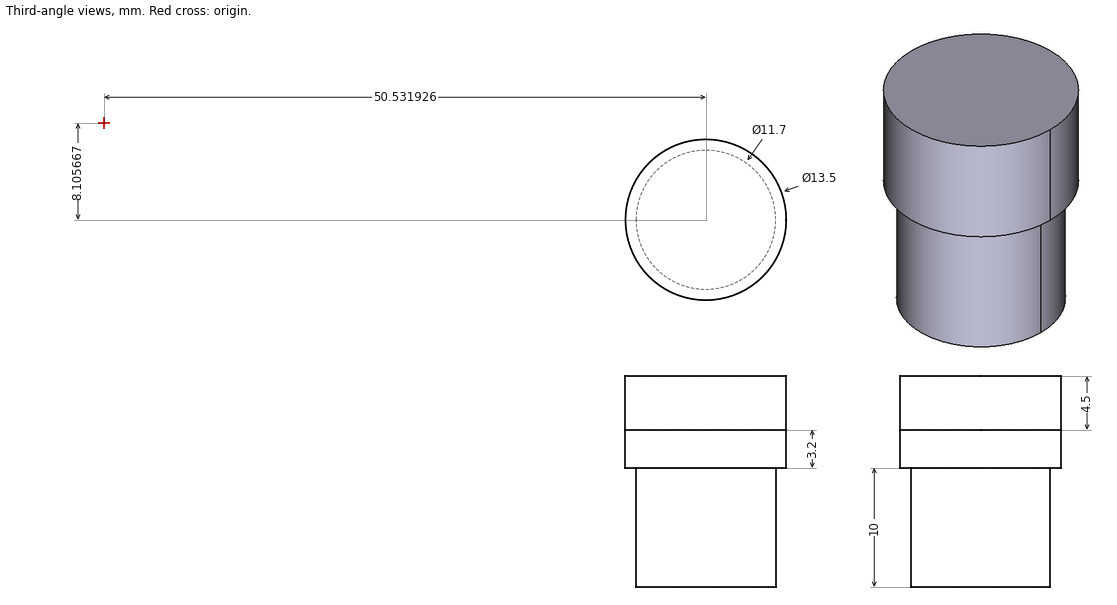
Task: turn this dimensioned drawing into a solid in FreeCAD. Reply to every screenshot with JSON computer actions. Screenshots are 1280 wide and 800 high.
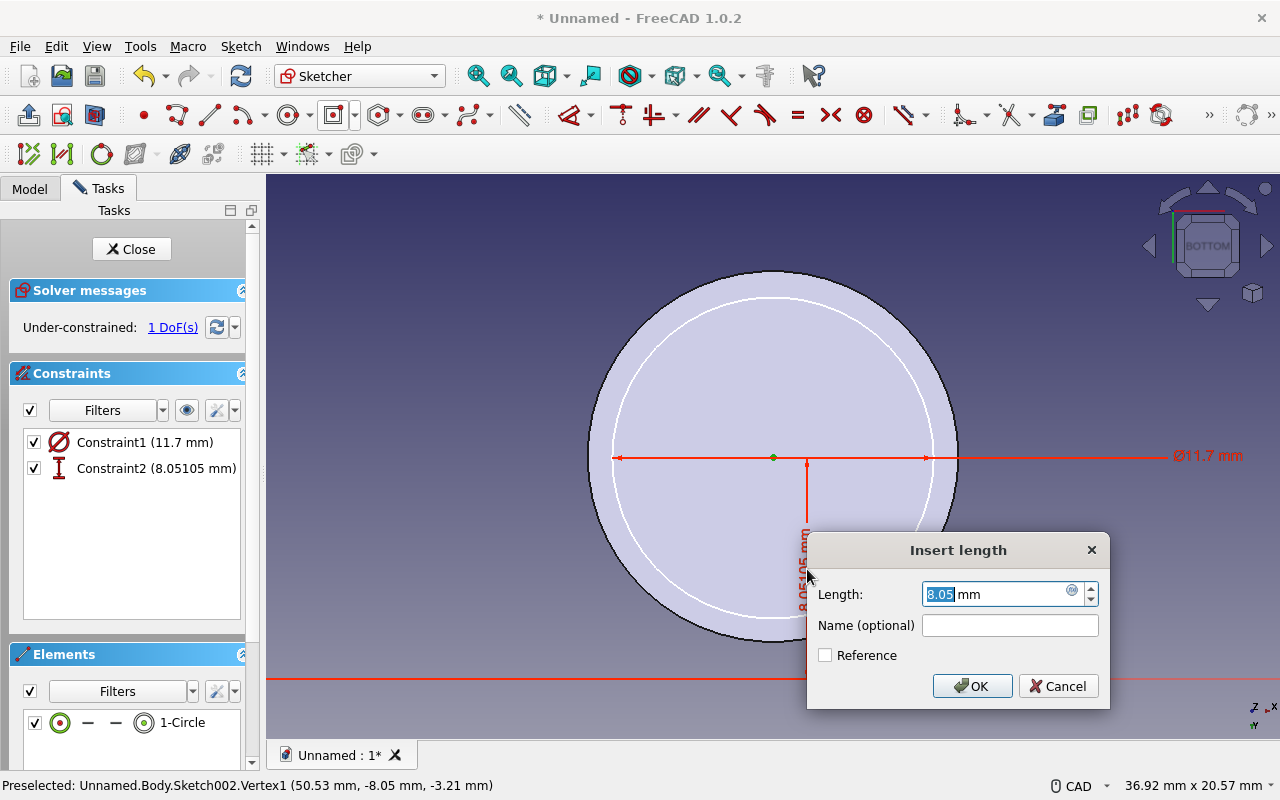
{"action": "type", "text": "8.105667"}
{"action": "key", "text": "Return"}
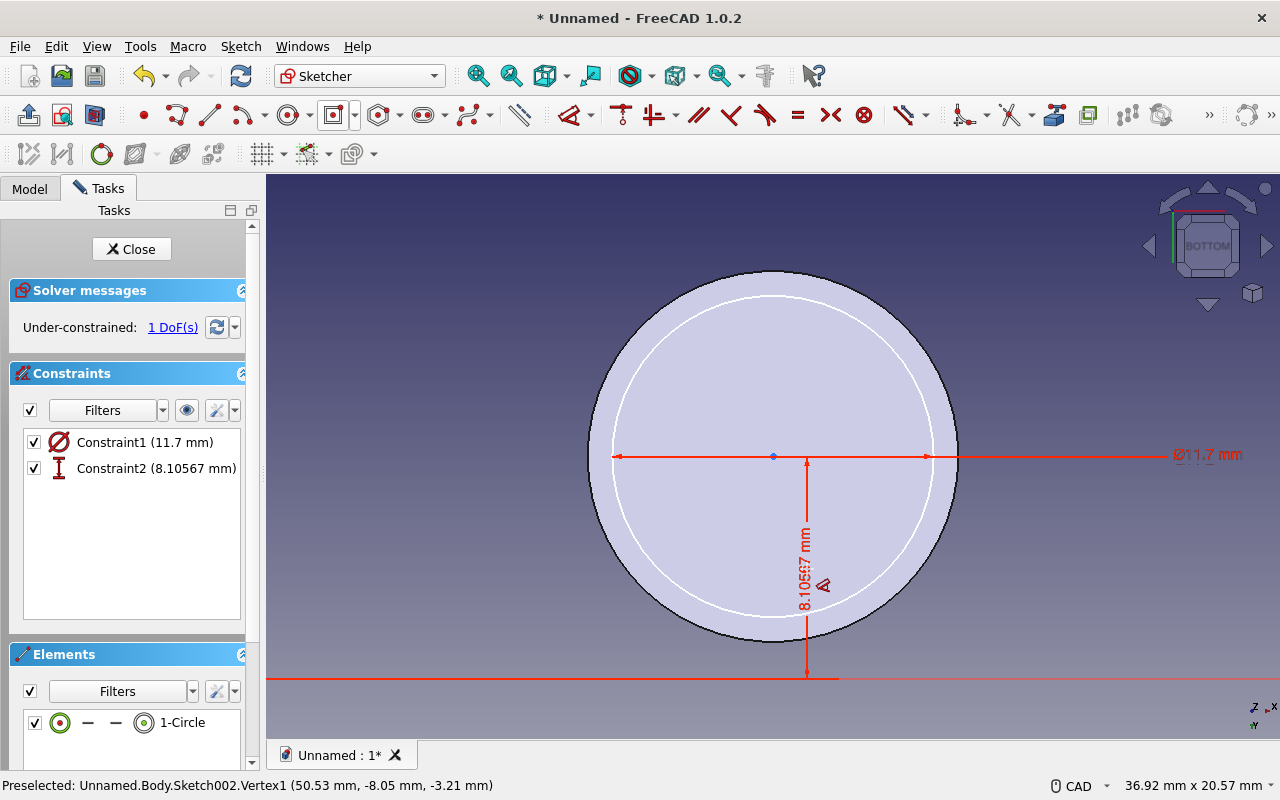
{"action": "left_click", "coordinate": [773, 457]}
{"action": "left_click", "coordinate": [533, 423]}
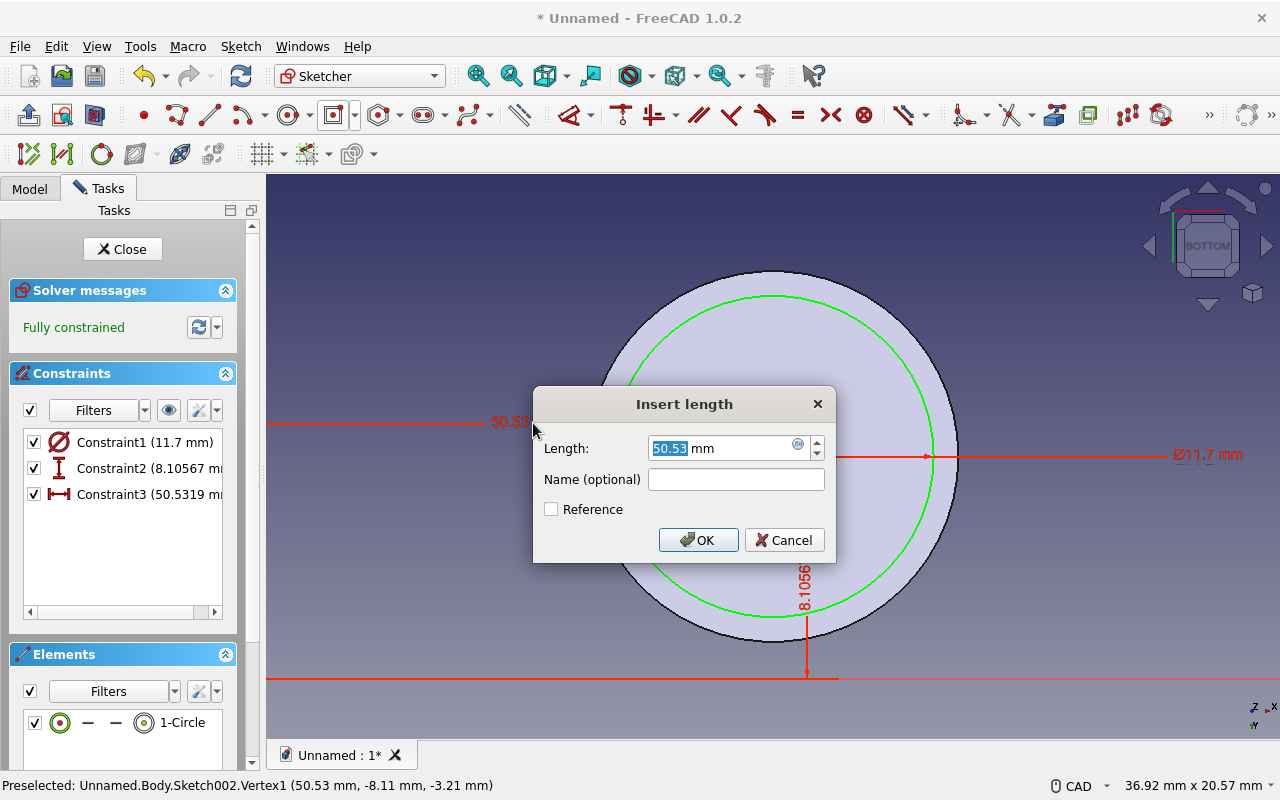
{"action": "type", "text": "50.531926"}
{"action": "key", "text": "Return"}
{"action": "key", "text": "Escape"}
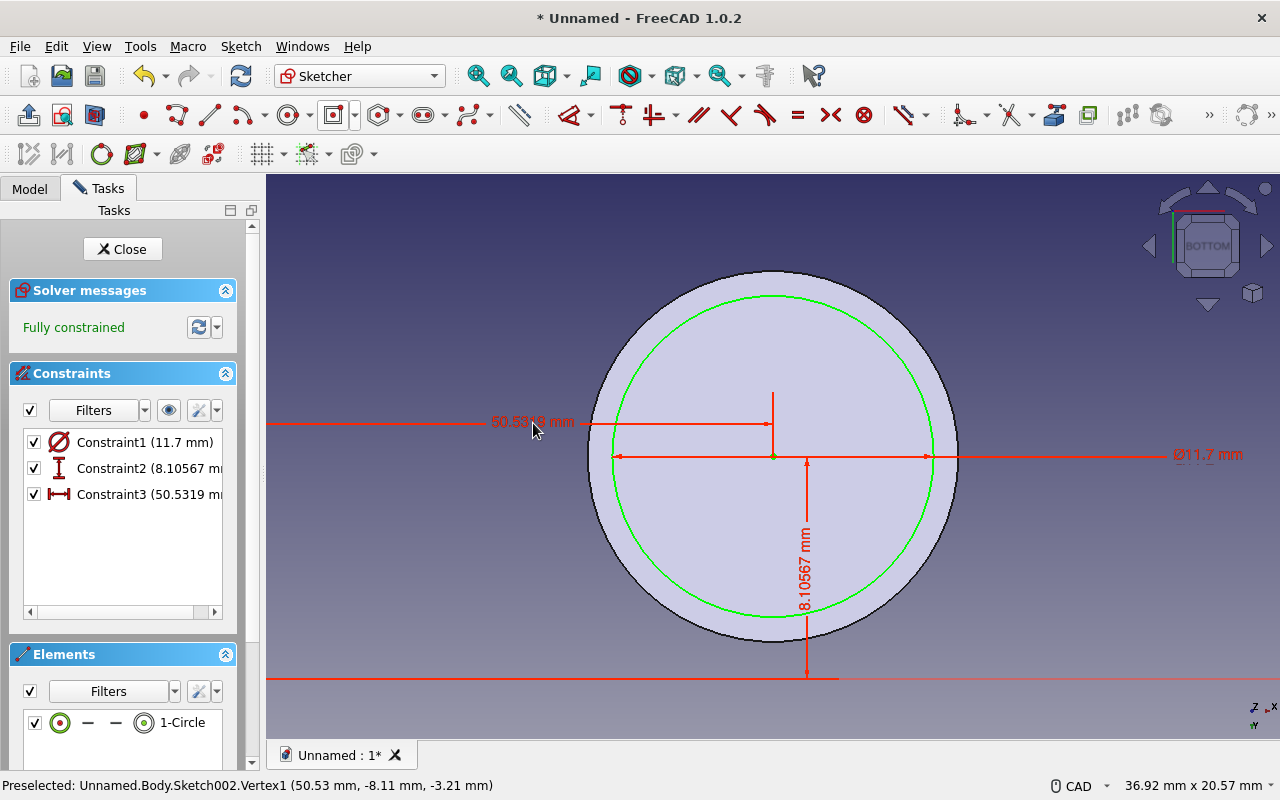
{"action": "left_click", "coordinate": [123, 249]}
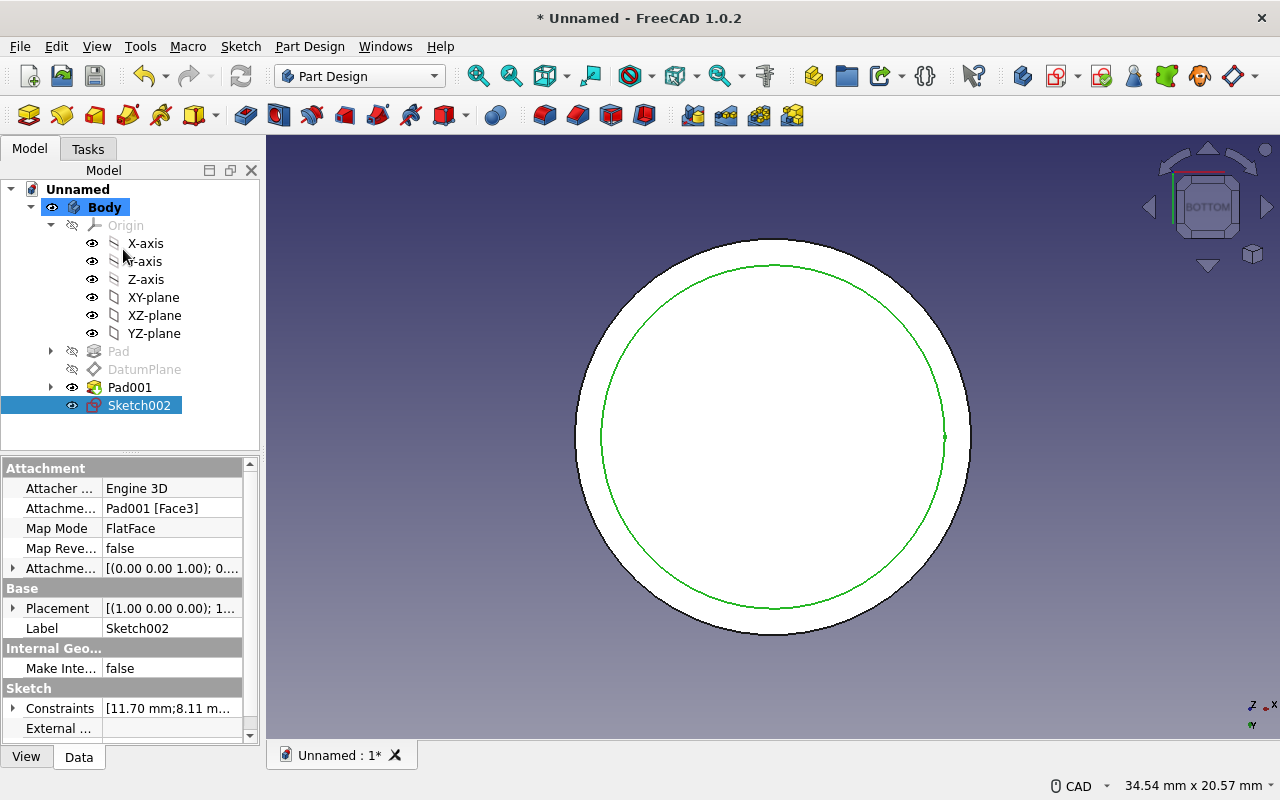
{"action": "left_click", "coordinate": [29, 116]}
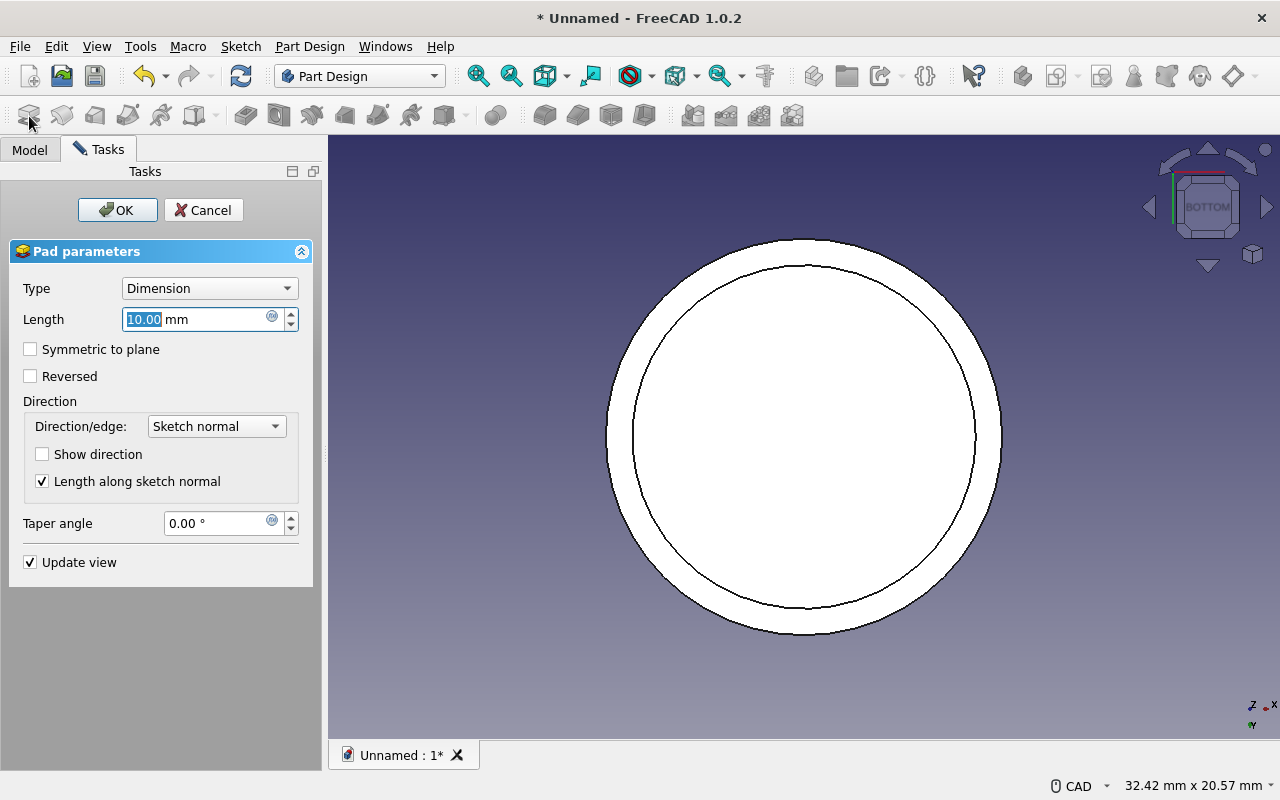
{"action": "type", "text": "10"}
{"action": "key", "text": "Tab"}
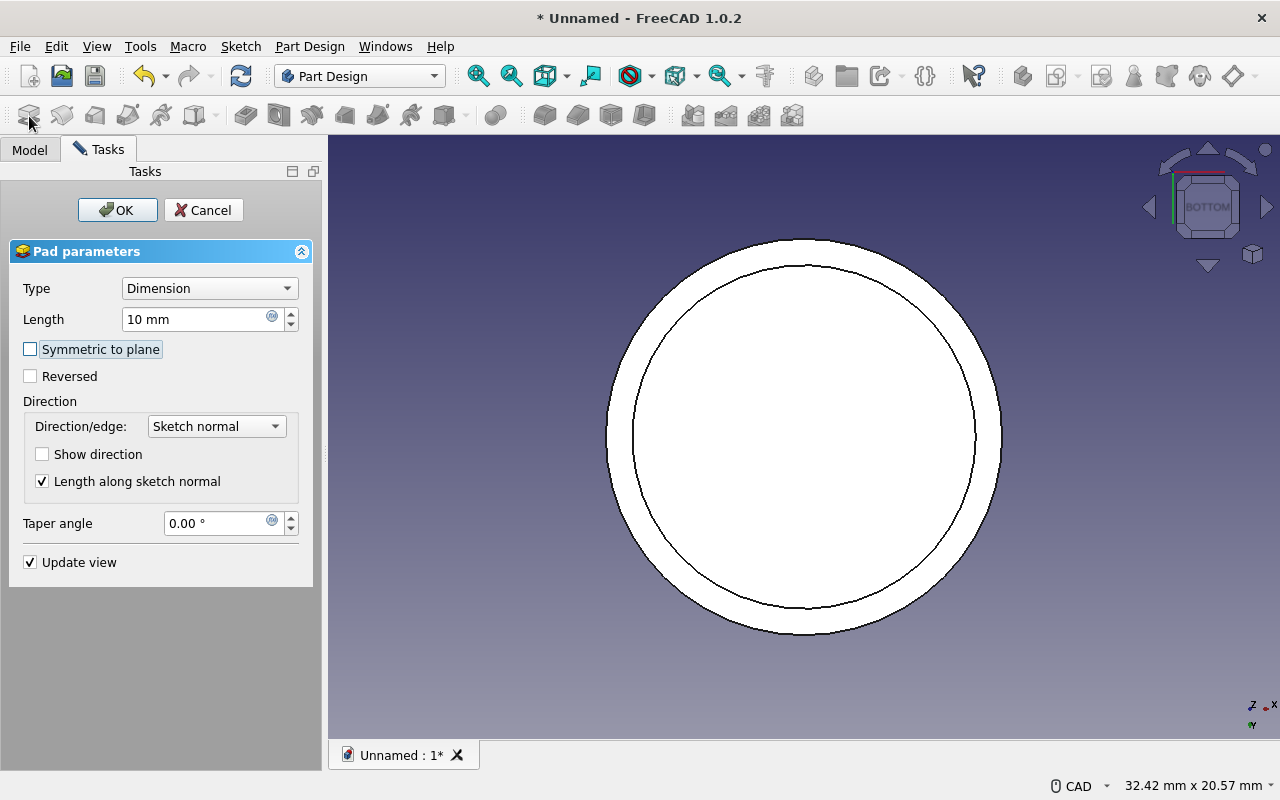
{"action": "left_click", "coordinate": [118, 210]}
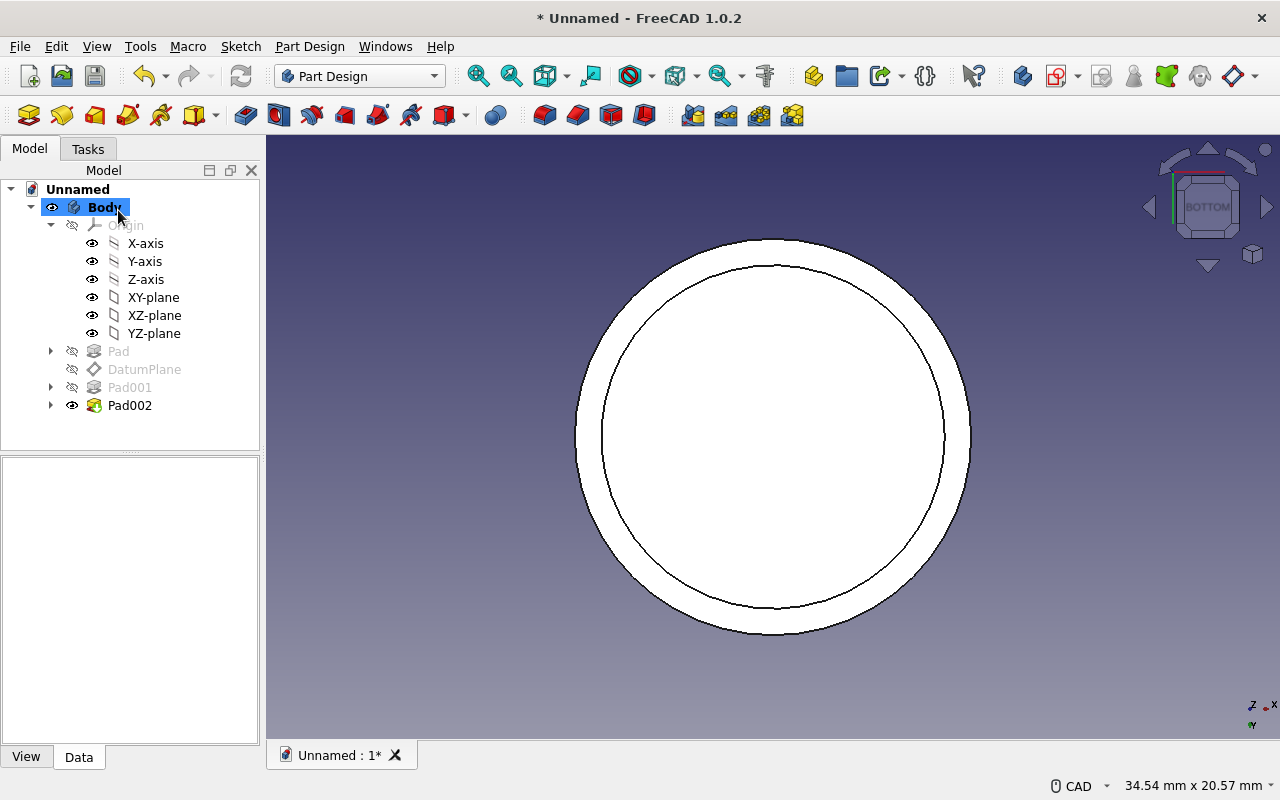
{"action": "key", "text": "0"}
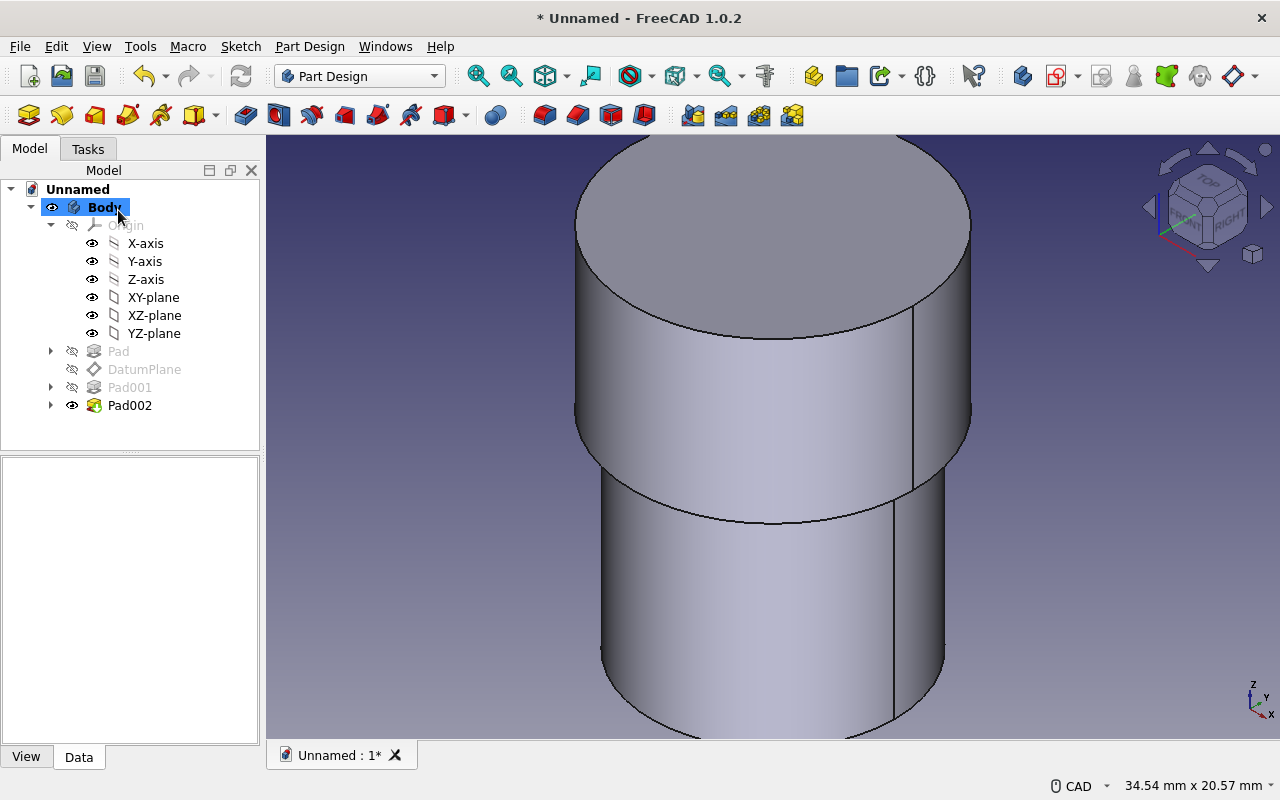
{"action": "key", "text": "v f"}